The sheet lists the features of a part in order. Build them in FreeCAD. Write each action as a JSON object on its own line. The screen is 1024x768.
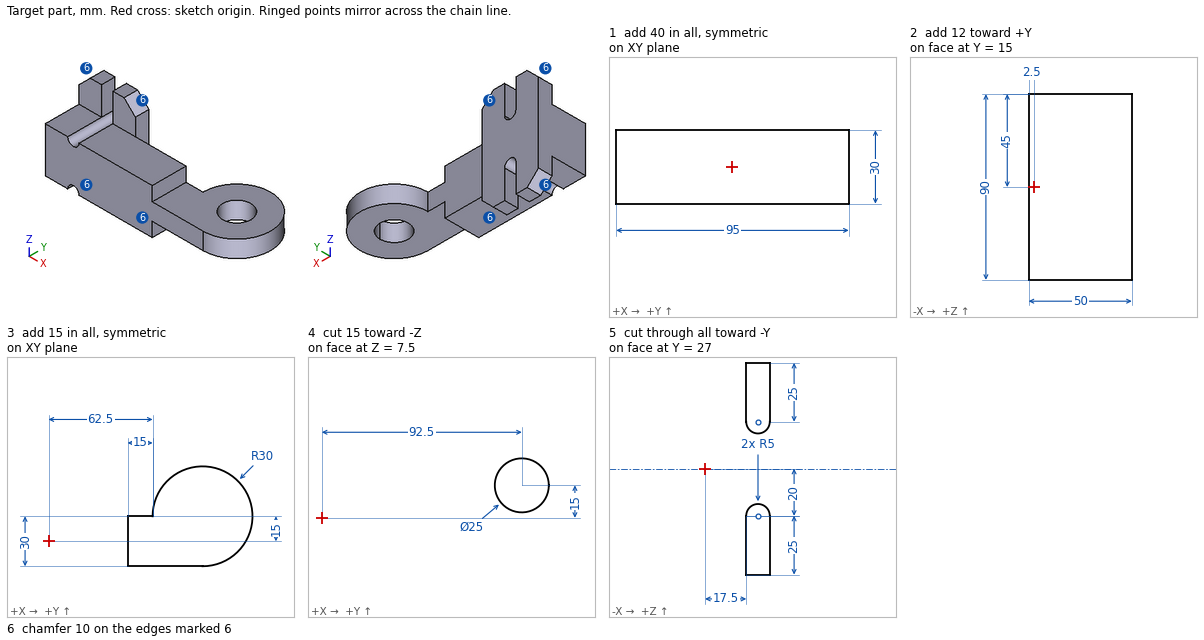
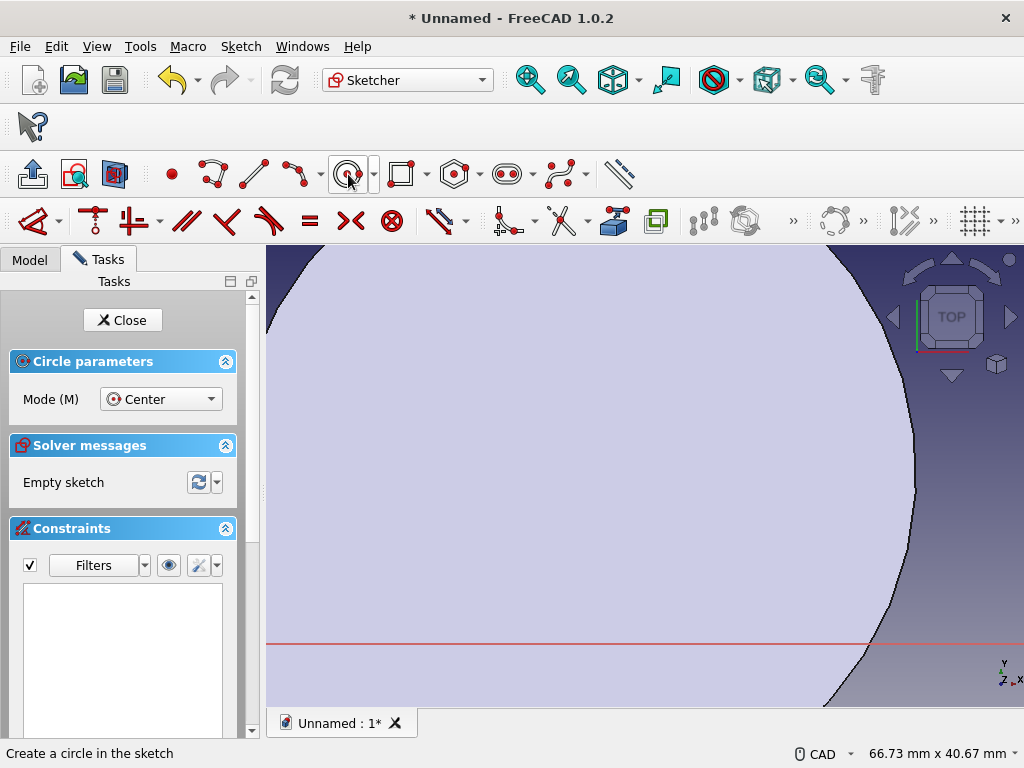
{"action": "left_click", "coordinate": [575, 474]}
{"action": "left_click", "coordinate": [676, 373]}
{"action": "key", "text": "Escape"}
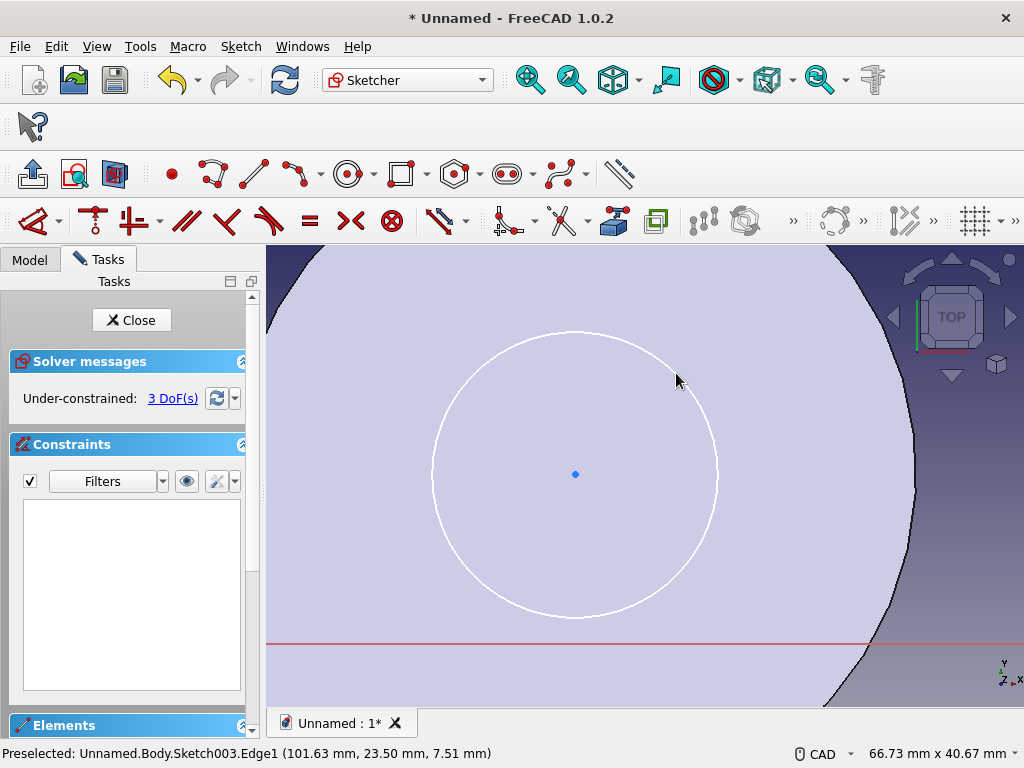
{"action": "key", "text": "d"}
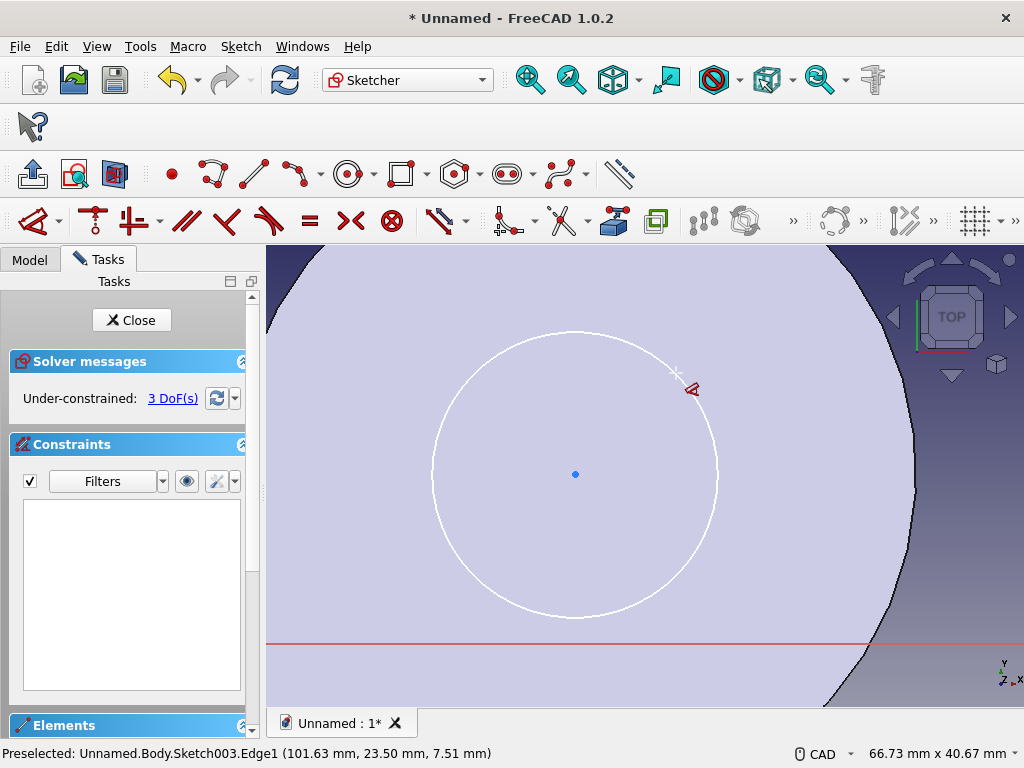
{"action": "left_click", "coordinate": [676, 374]}
{"action": "left_click", "coordinate": [699, 351]}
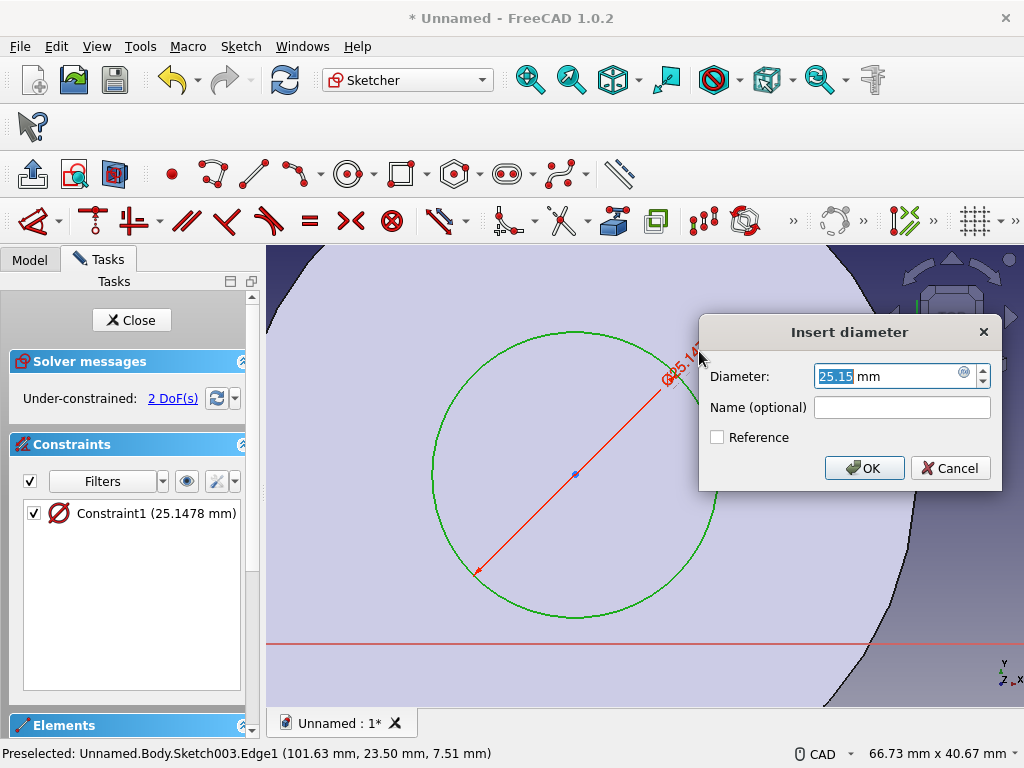
{"action": "type", "text": "25"}
{"action": "key", "text": "Return"}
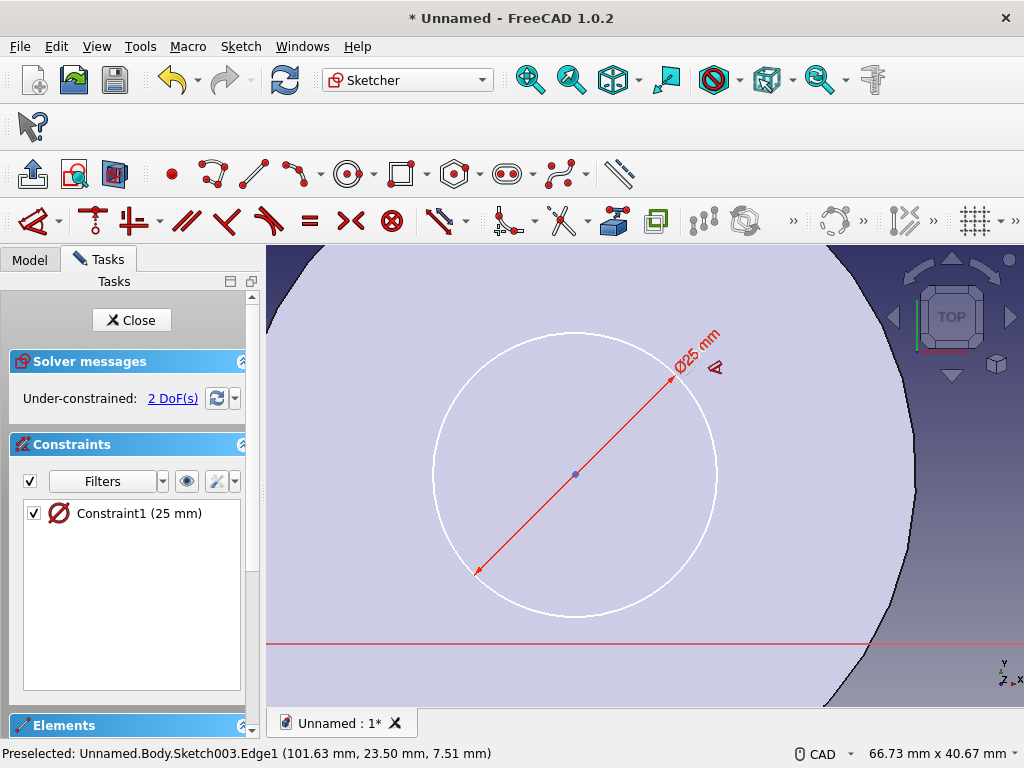
{"action": "left_click", "coordinate": [575, 475]}
{"action": "left_click", "coordinate": [609, 560]}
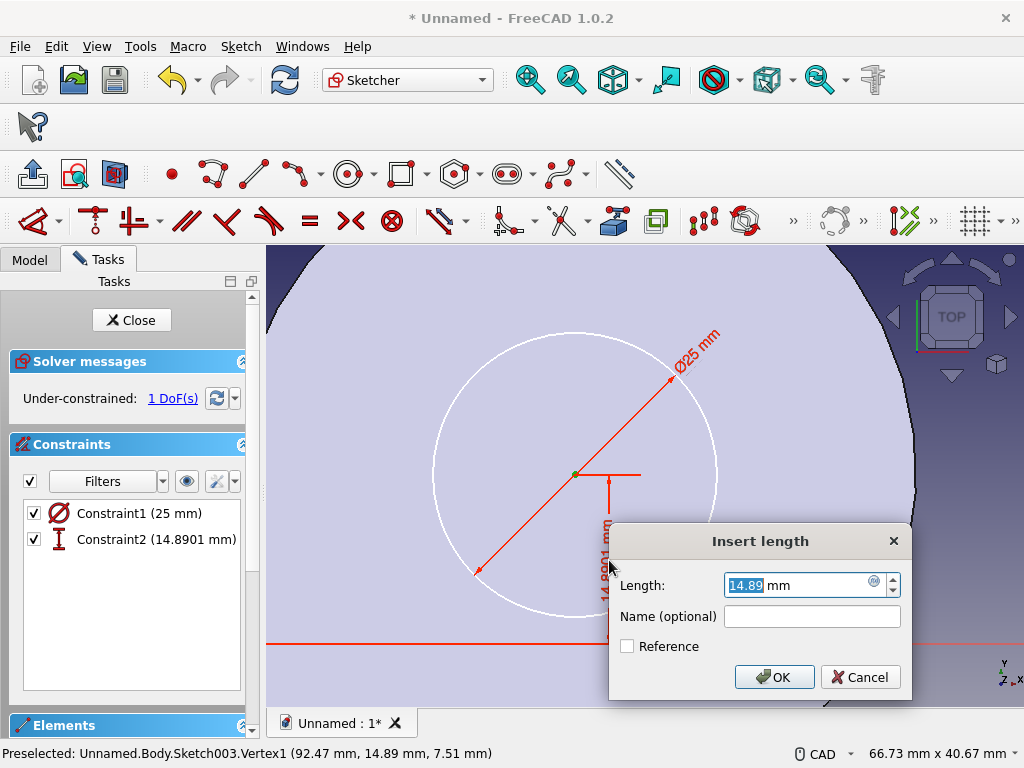
{"action": "type", "text": "15"}
{"action": "key", "text": "Return"}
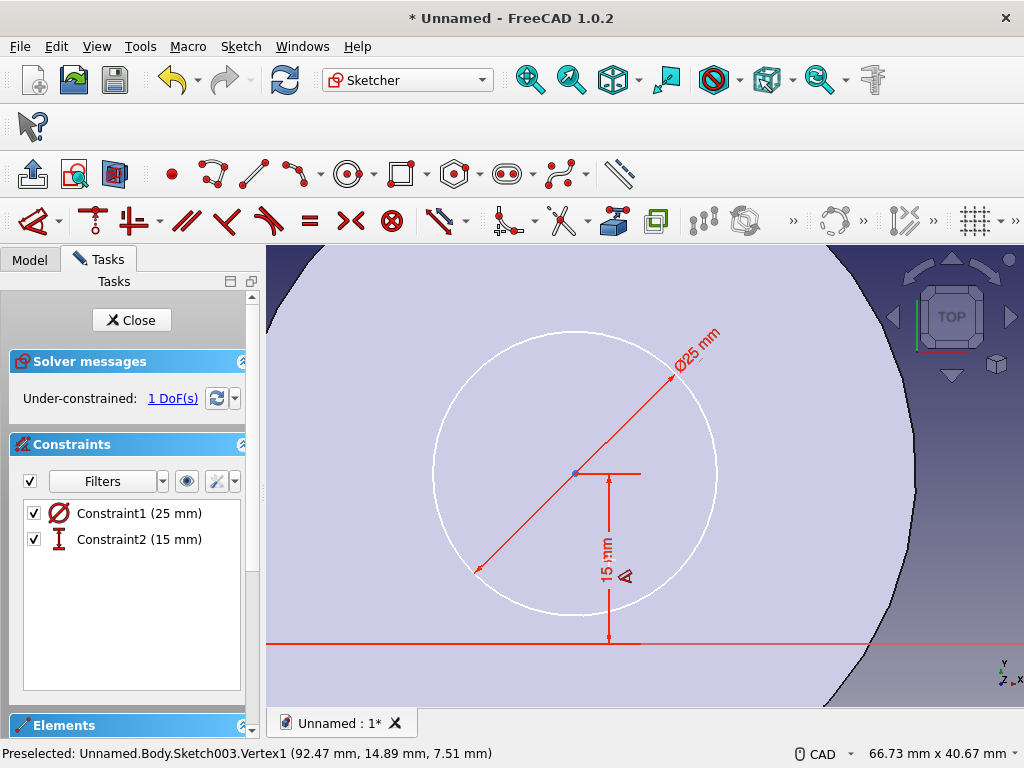
{"action": "left_click", "coordinate": [575, 474]}
{"action": "left_click", "coordinate": [434, 678]}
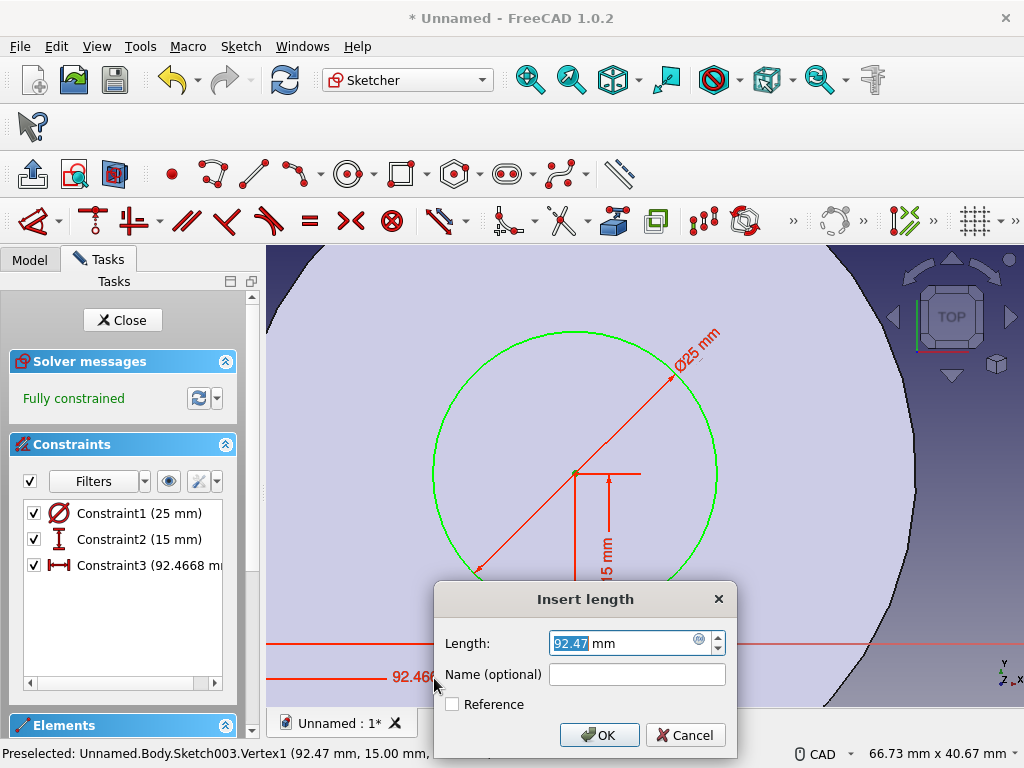
{"action": "type", "text": "92.5"}
{"action": "key", "text": "Return"}
{"action": "key", "text": "Escape"}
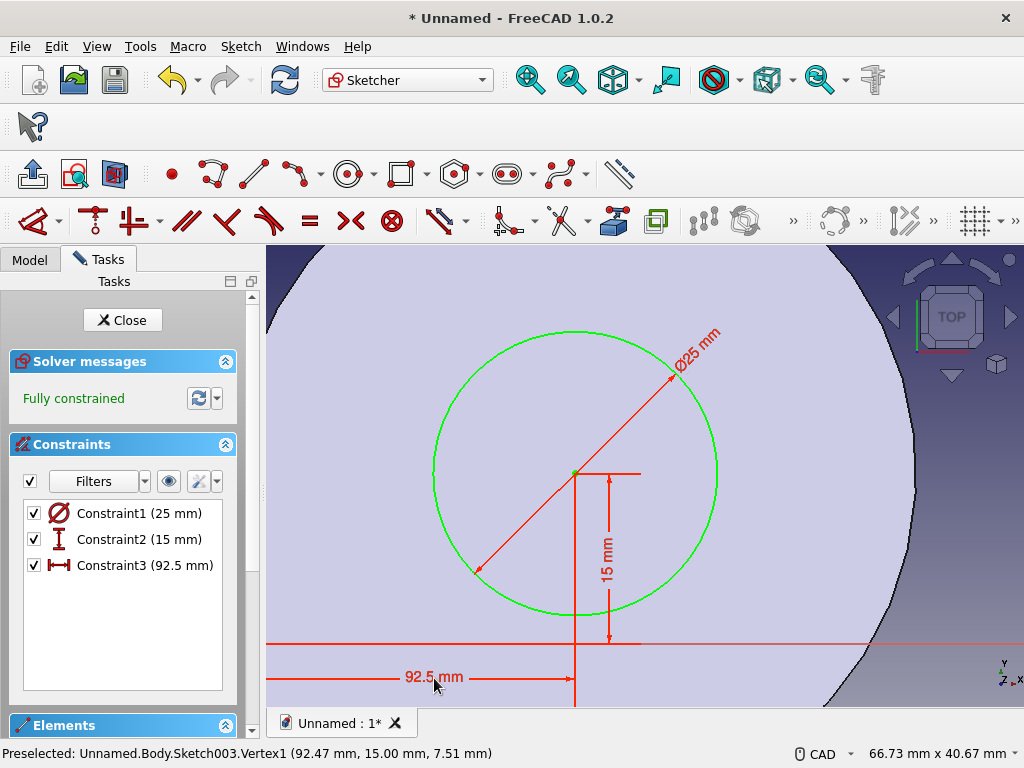
{"action": "left_click", "coordinate": [123, 320]}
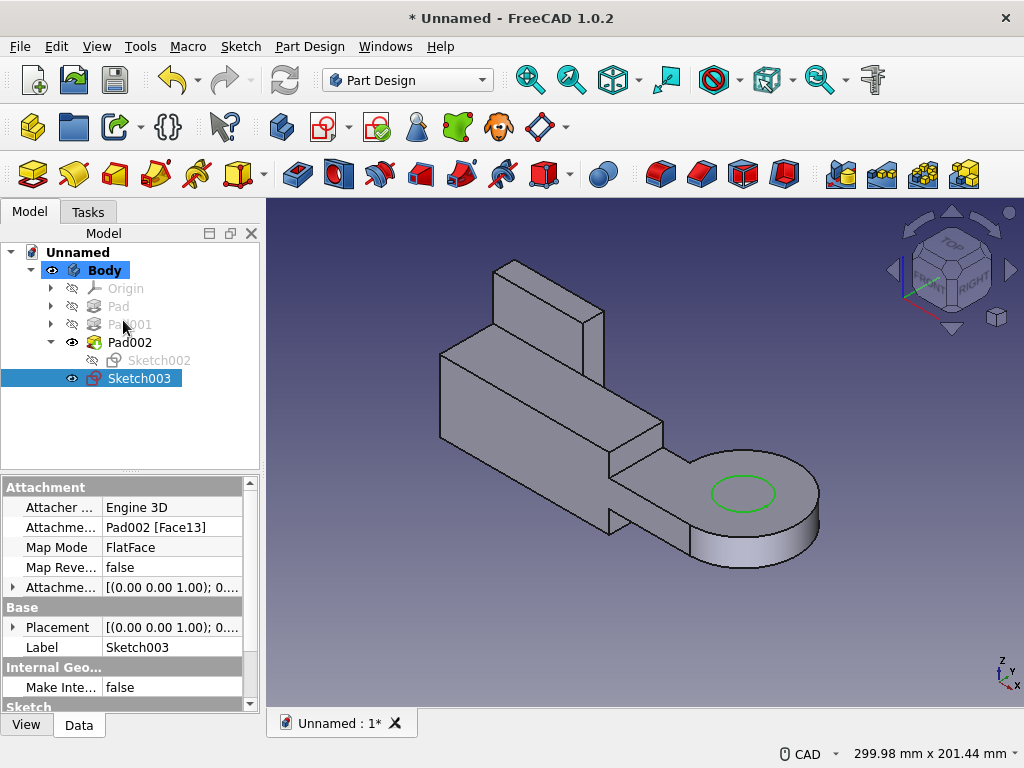
{"action": "left_click", "coordinate": [298, 174]}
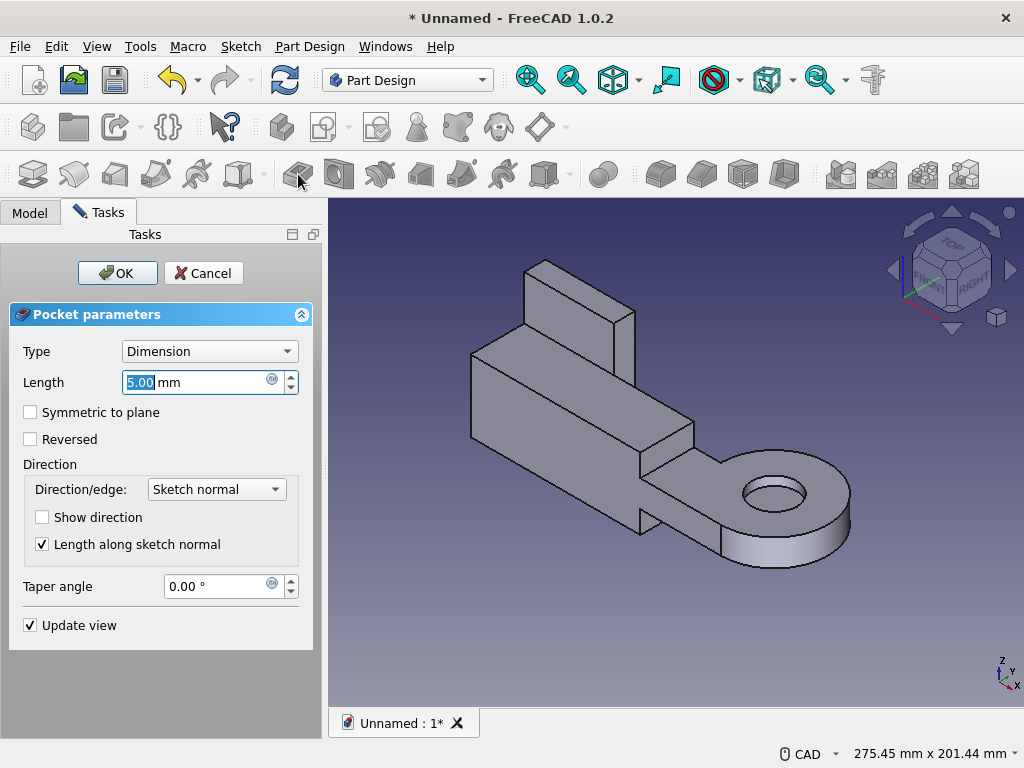
{"action": "type", "text": "15"}
{"action": "key", "text": "Tab"}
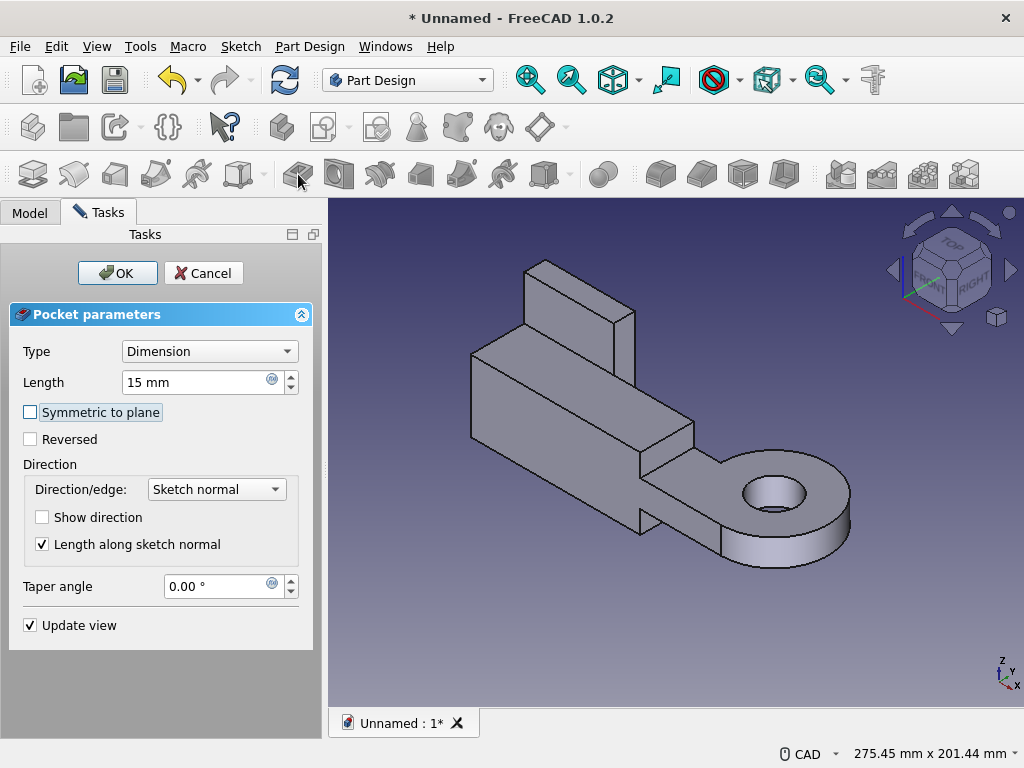
{"action": "left_click", "coordinate": [118, 273]}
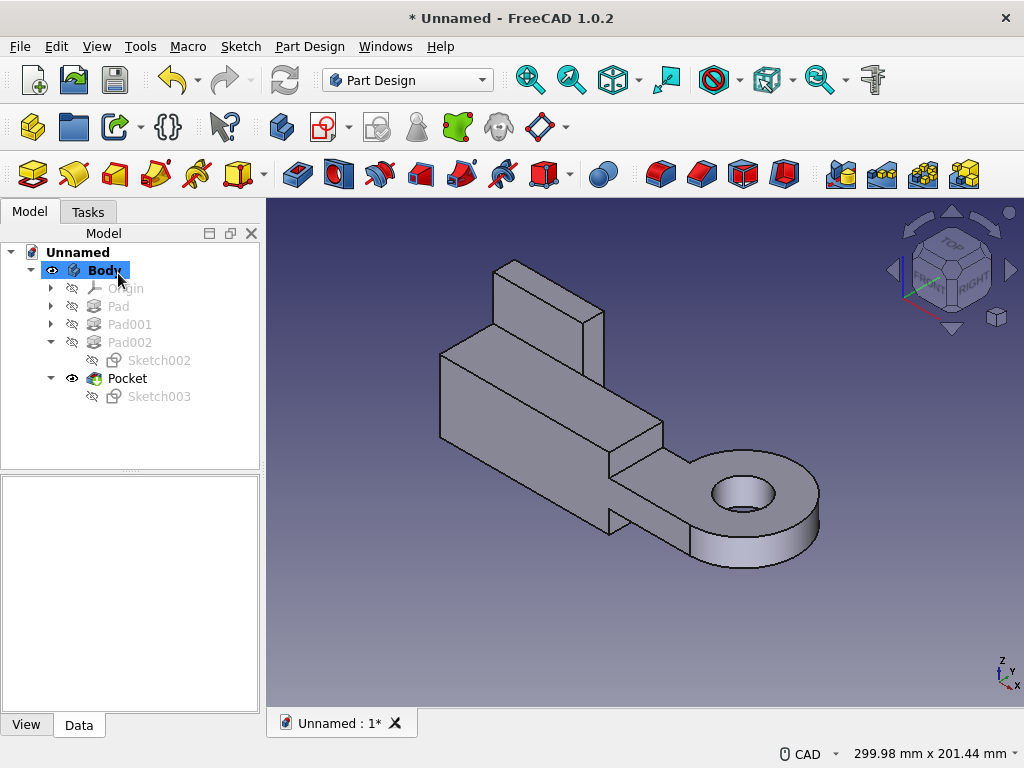
{"action": "key", "text": "4"}